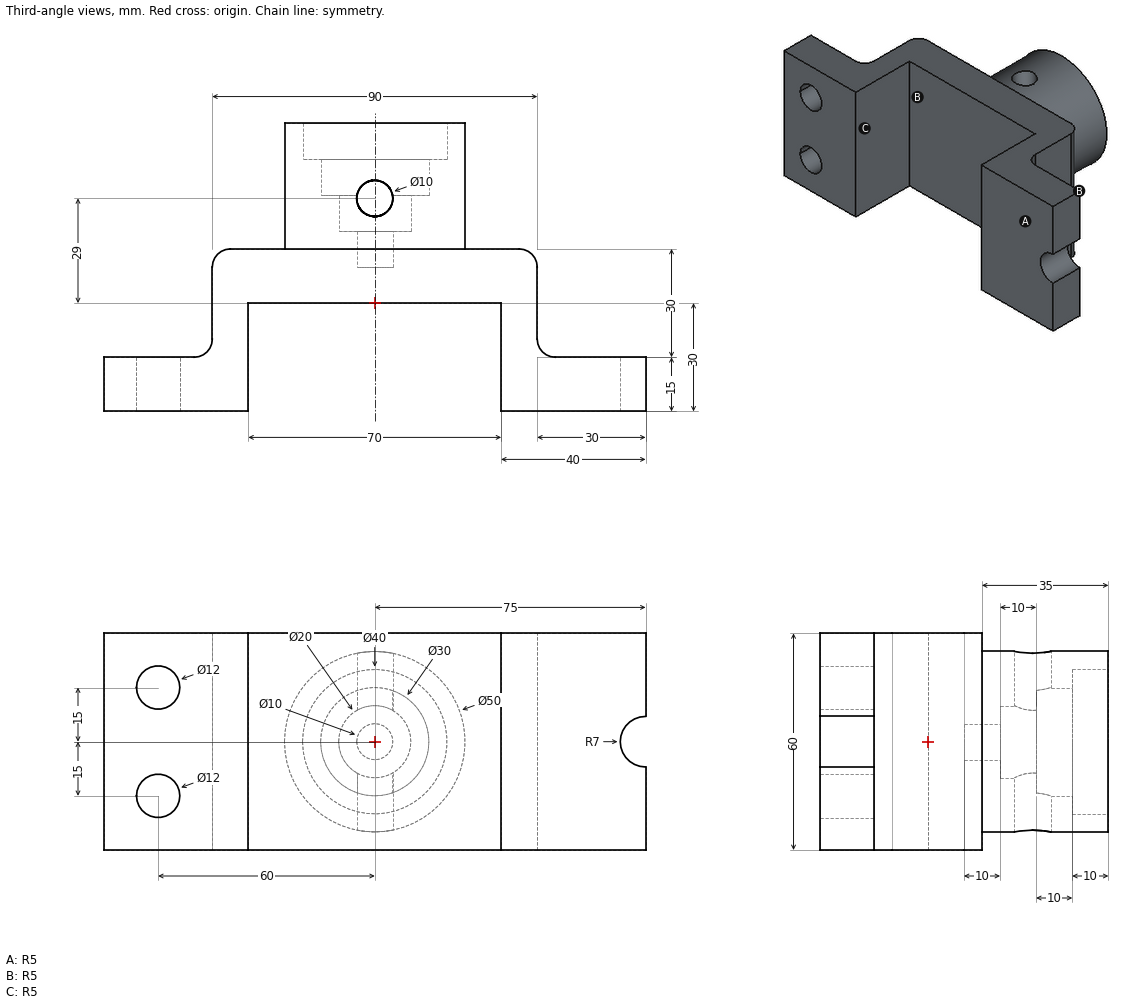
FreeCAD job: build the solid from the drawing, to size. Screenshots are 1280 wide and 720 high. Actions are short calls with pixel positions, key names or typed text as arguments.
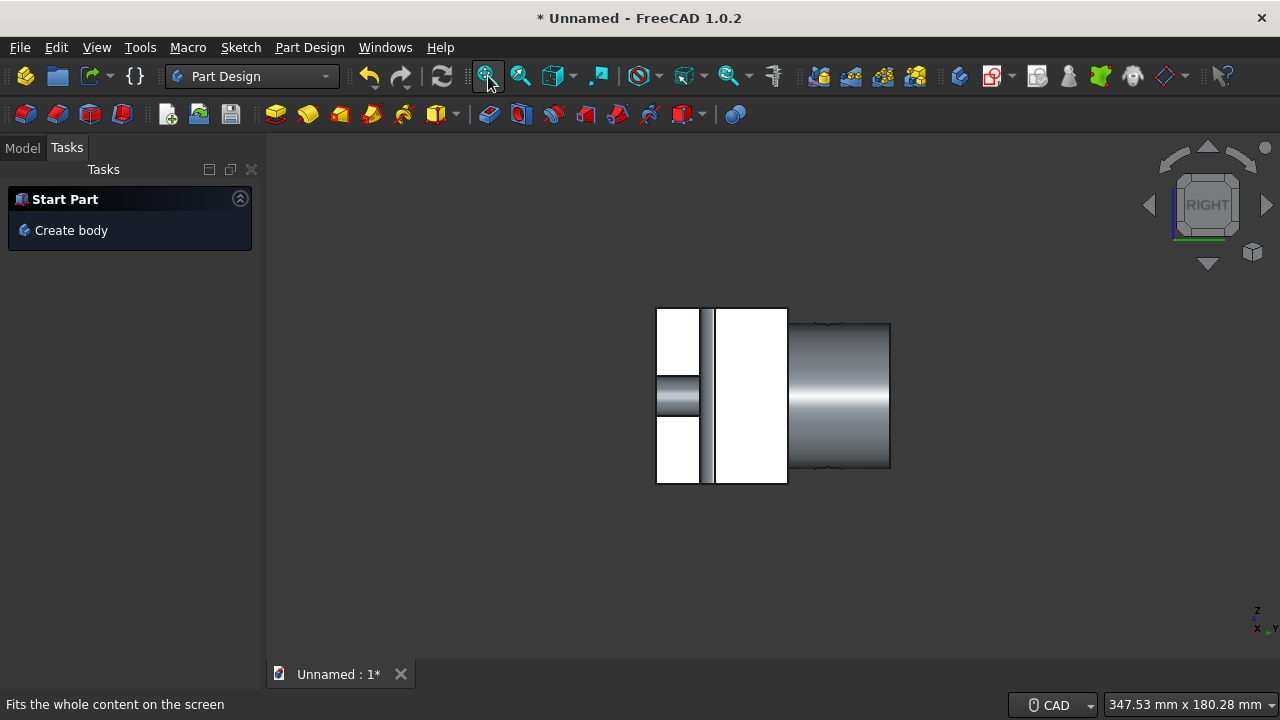
key(v)
key(f)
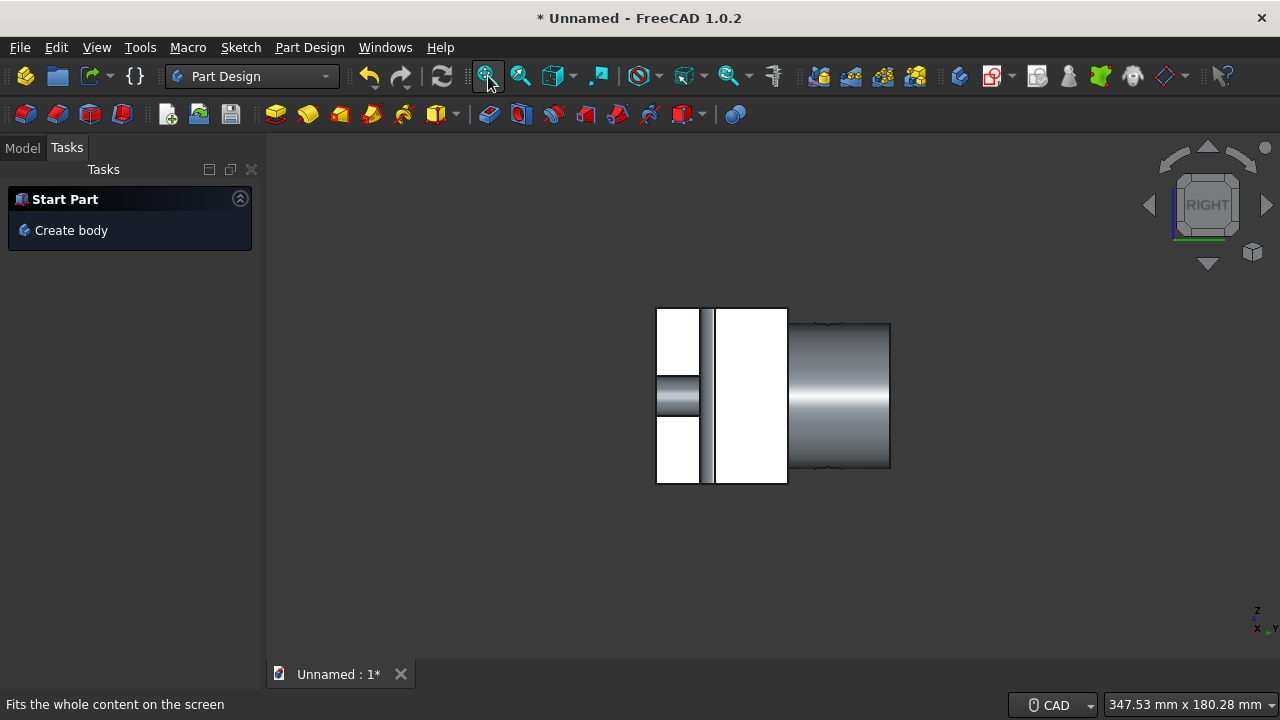
click(788, 395)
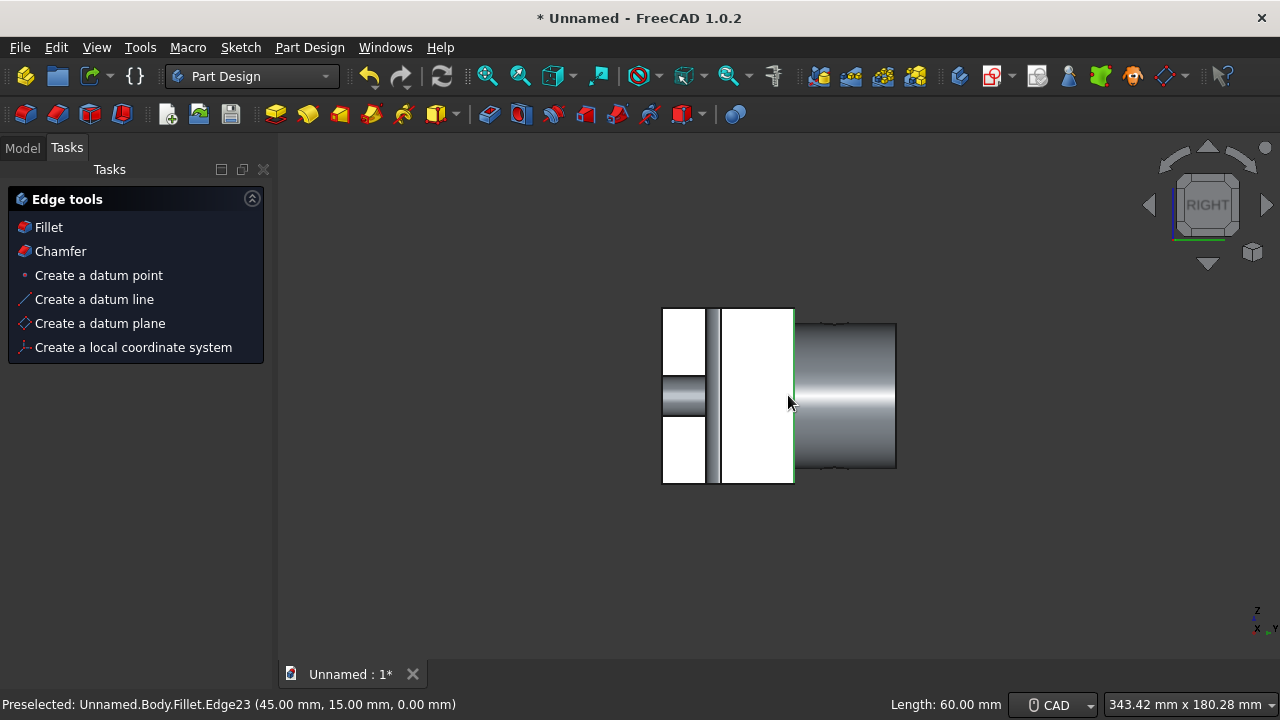
key(5)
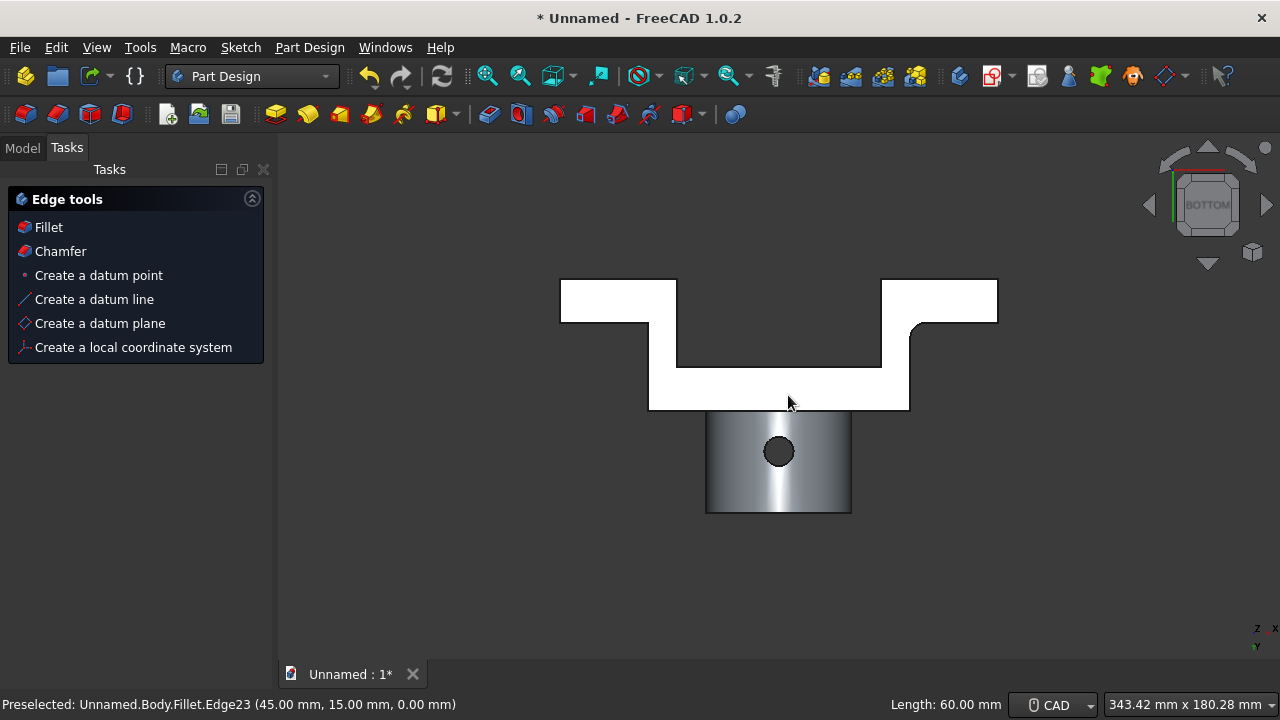
click(488, 76)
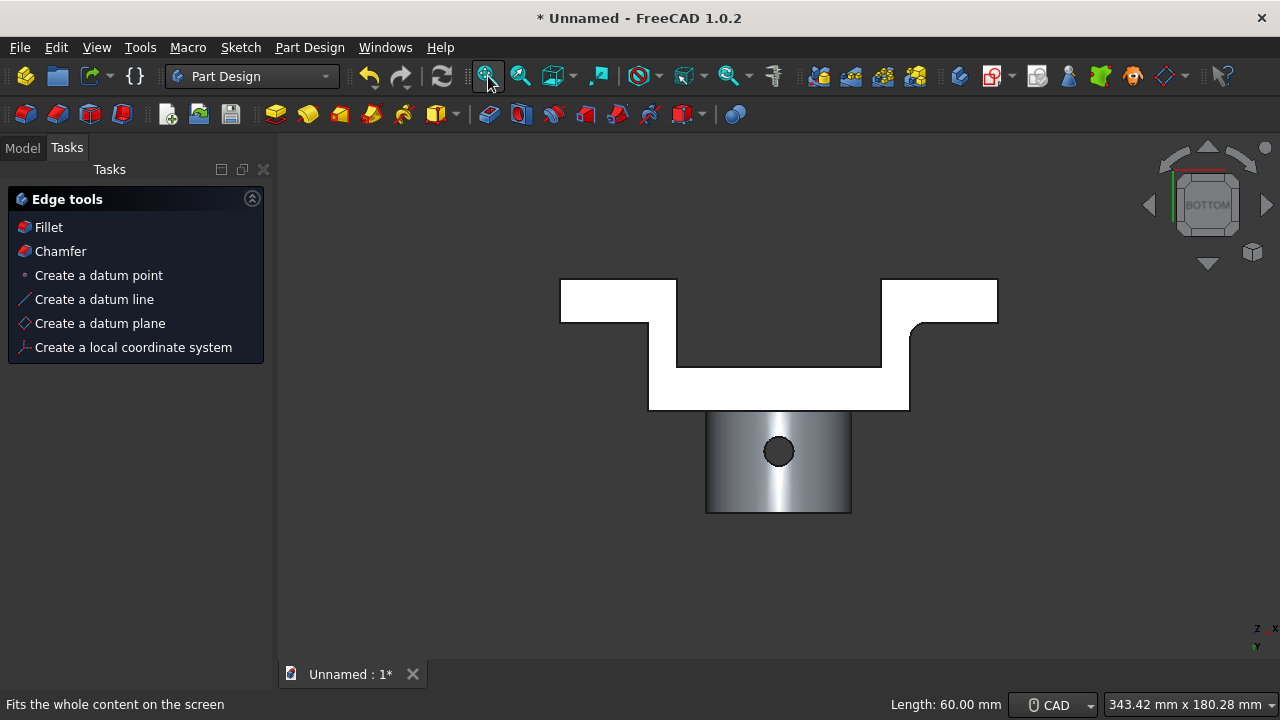
key(4)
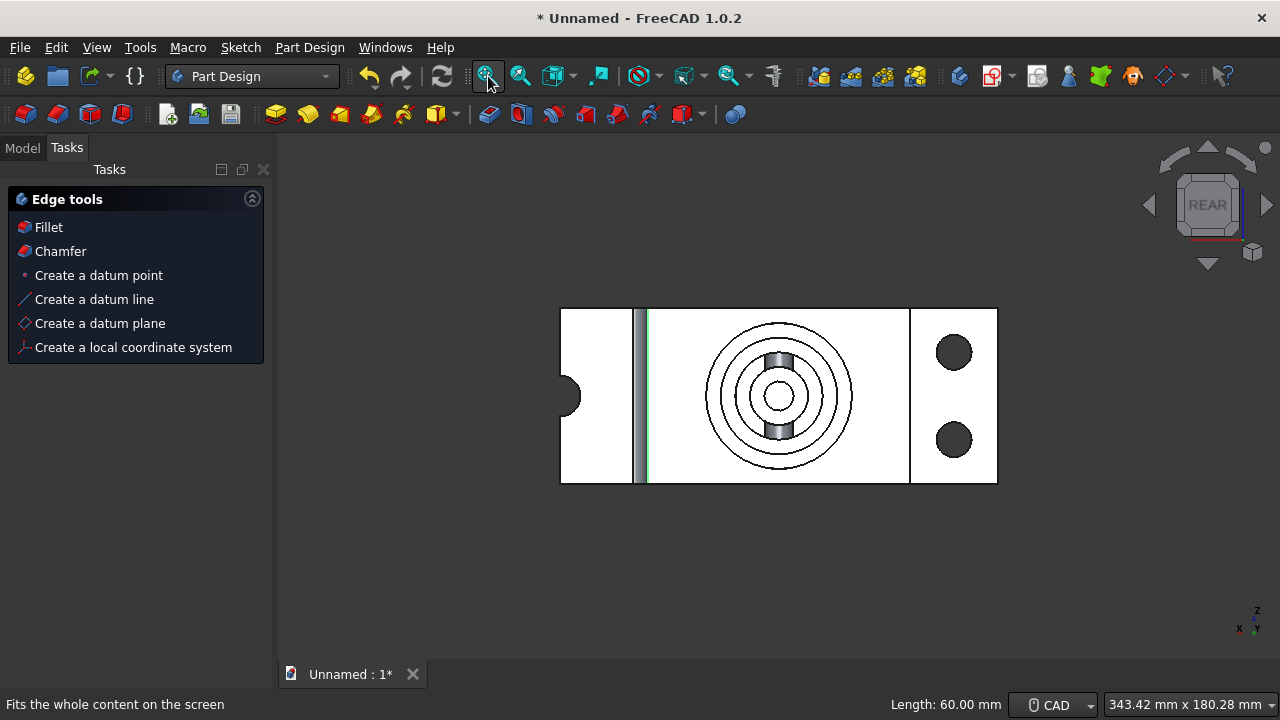
click(488, 76)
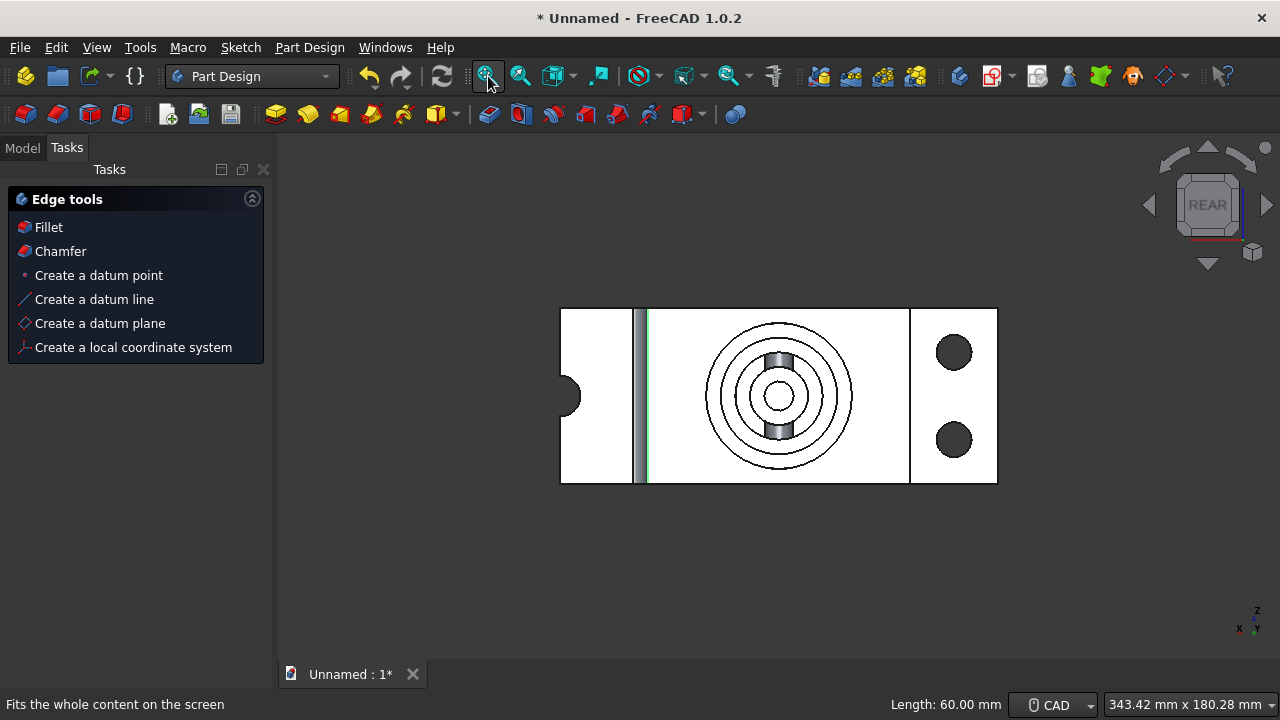
click(910, 395, ctrl)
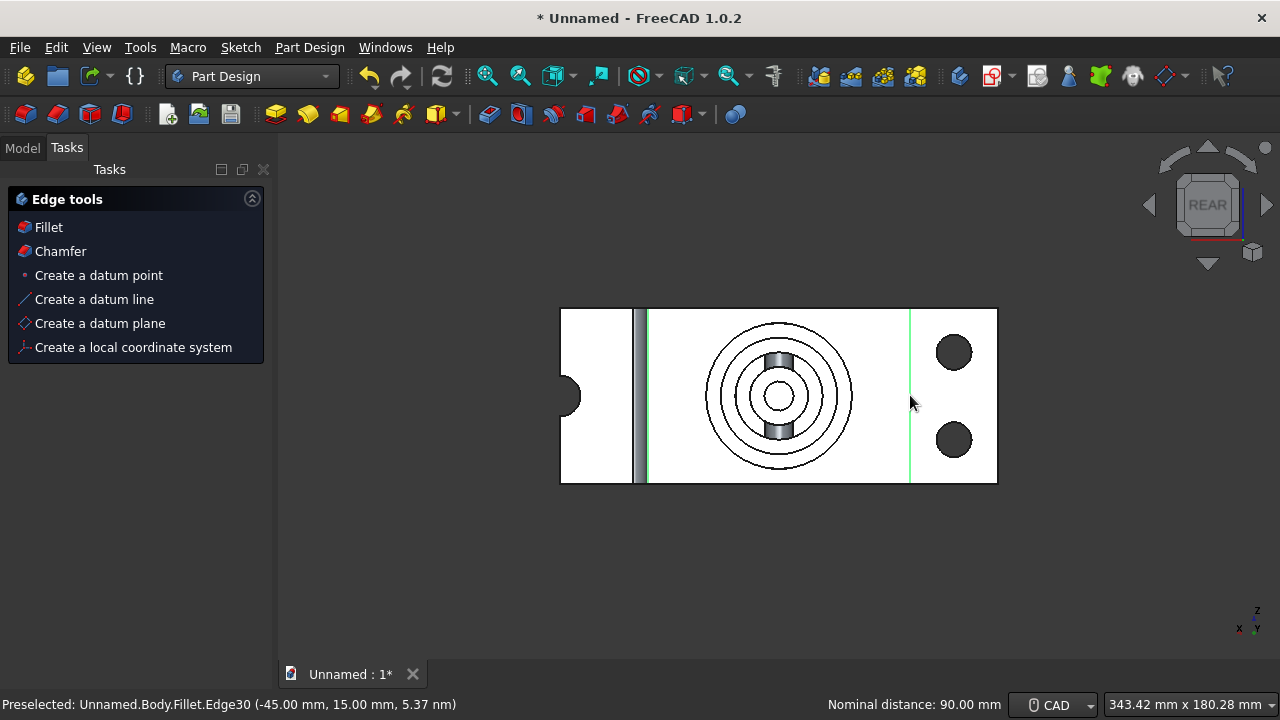
click(26, 114)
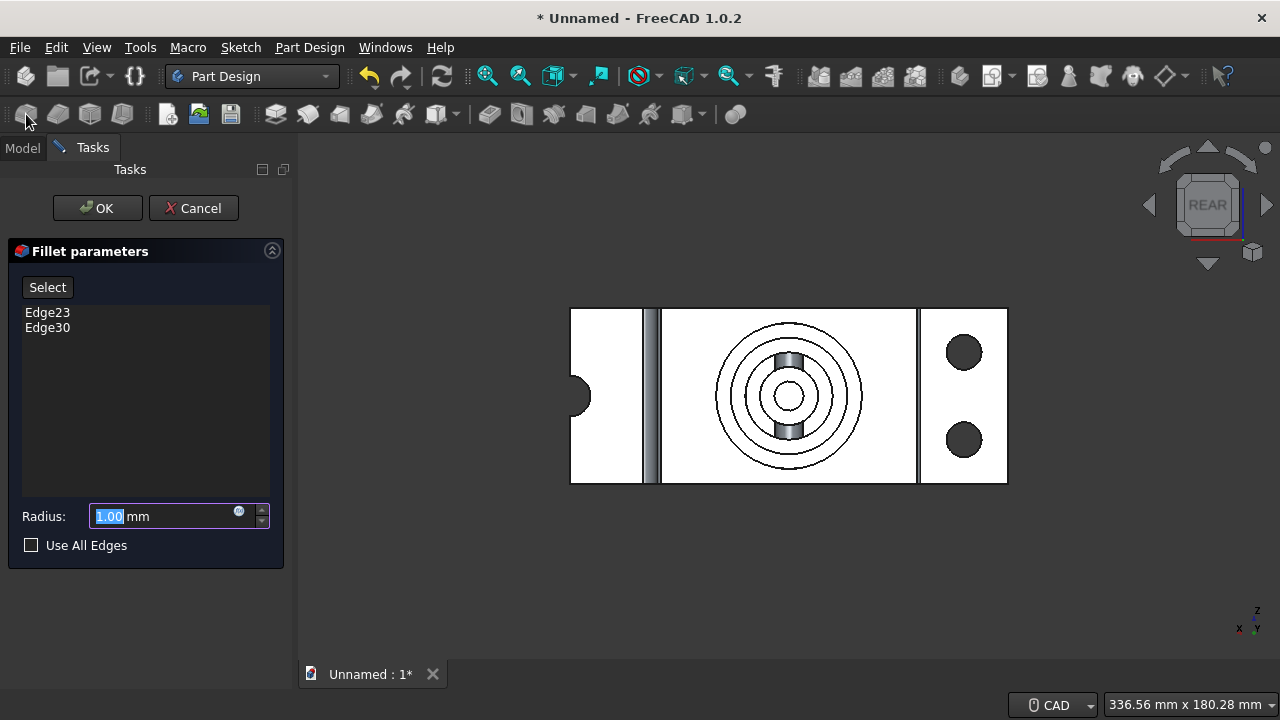
text(5)
key(Tab)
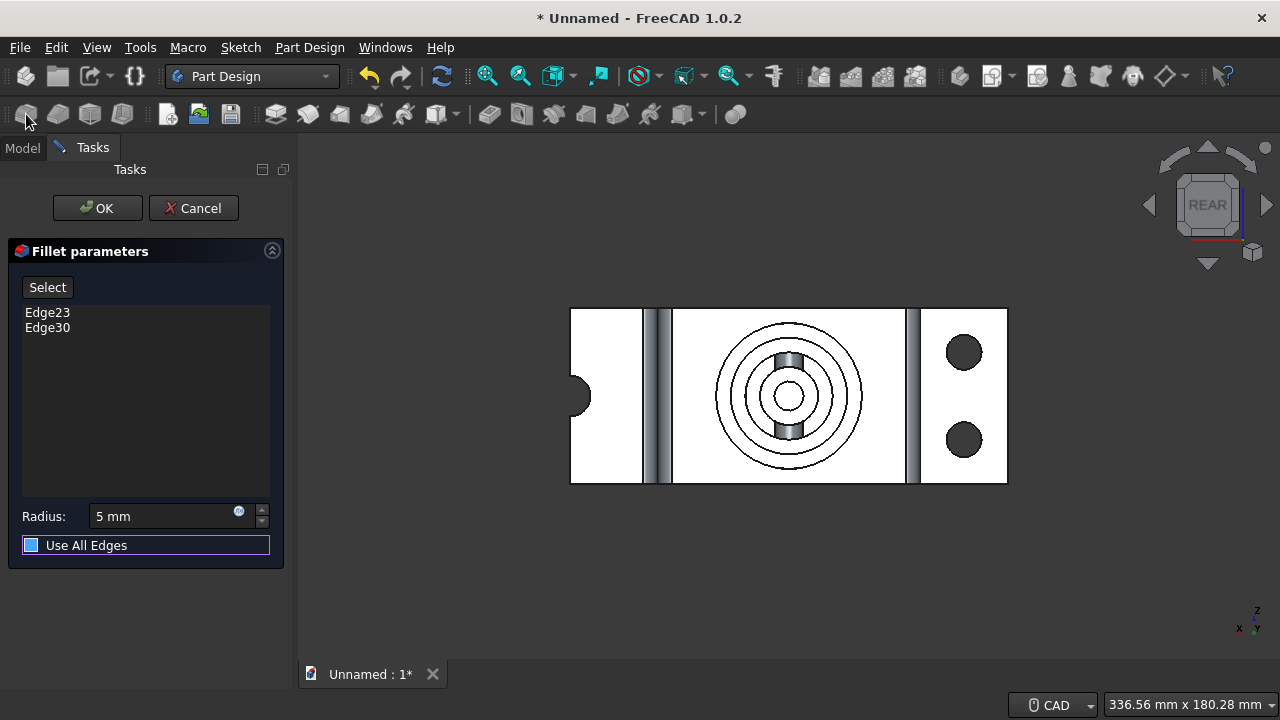
click(98, 208)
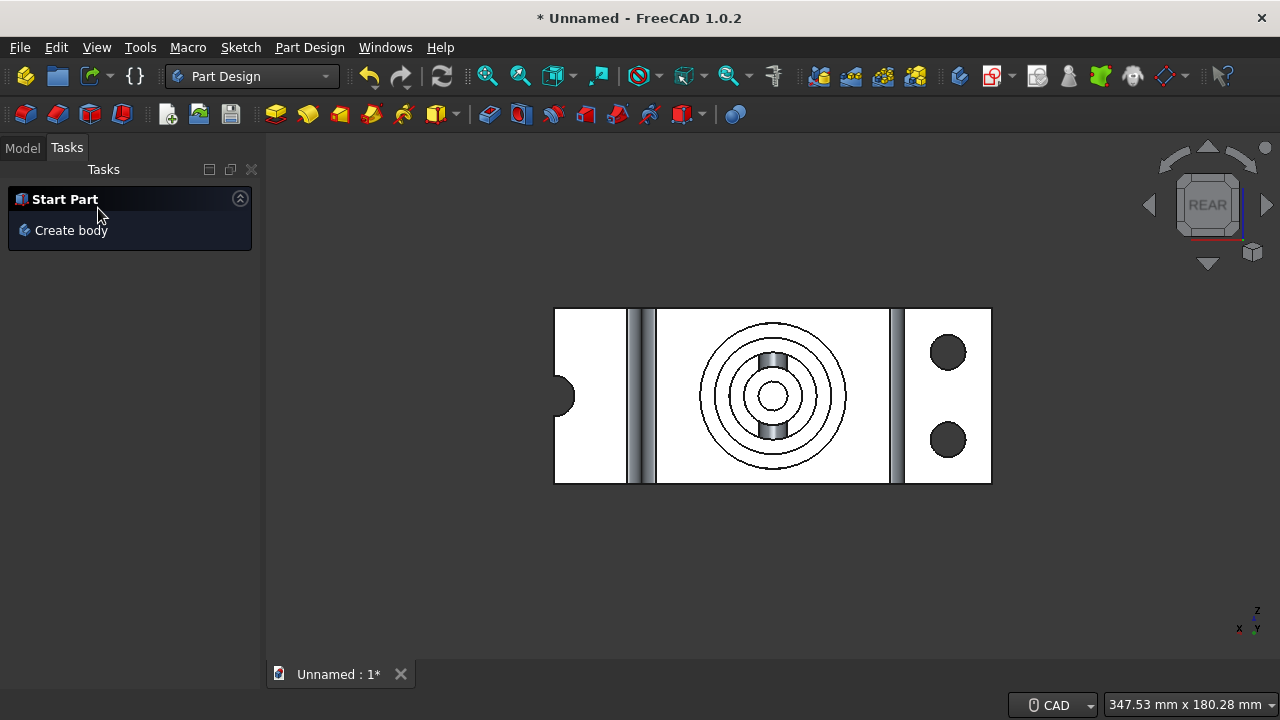
click(488, 76)